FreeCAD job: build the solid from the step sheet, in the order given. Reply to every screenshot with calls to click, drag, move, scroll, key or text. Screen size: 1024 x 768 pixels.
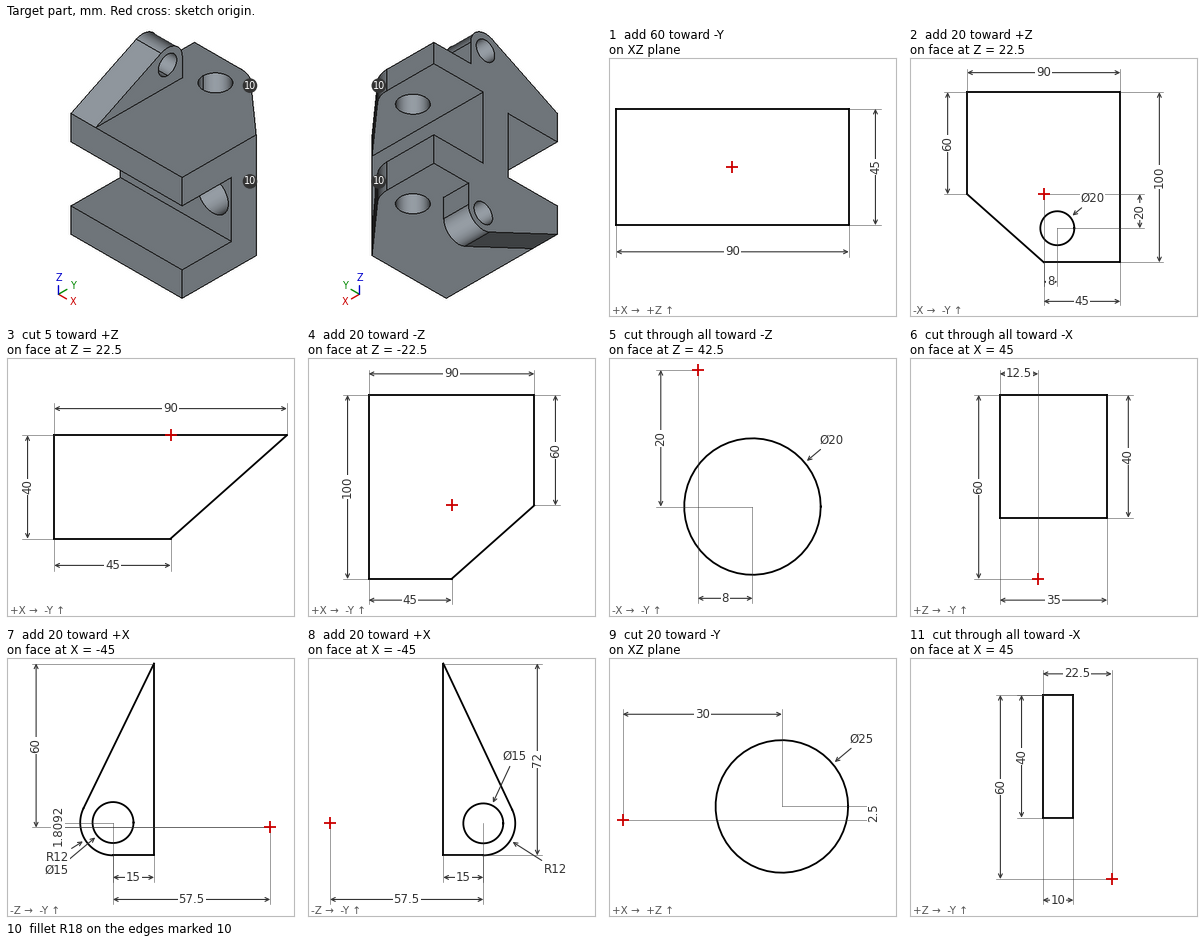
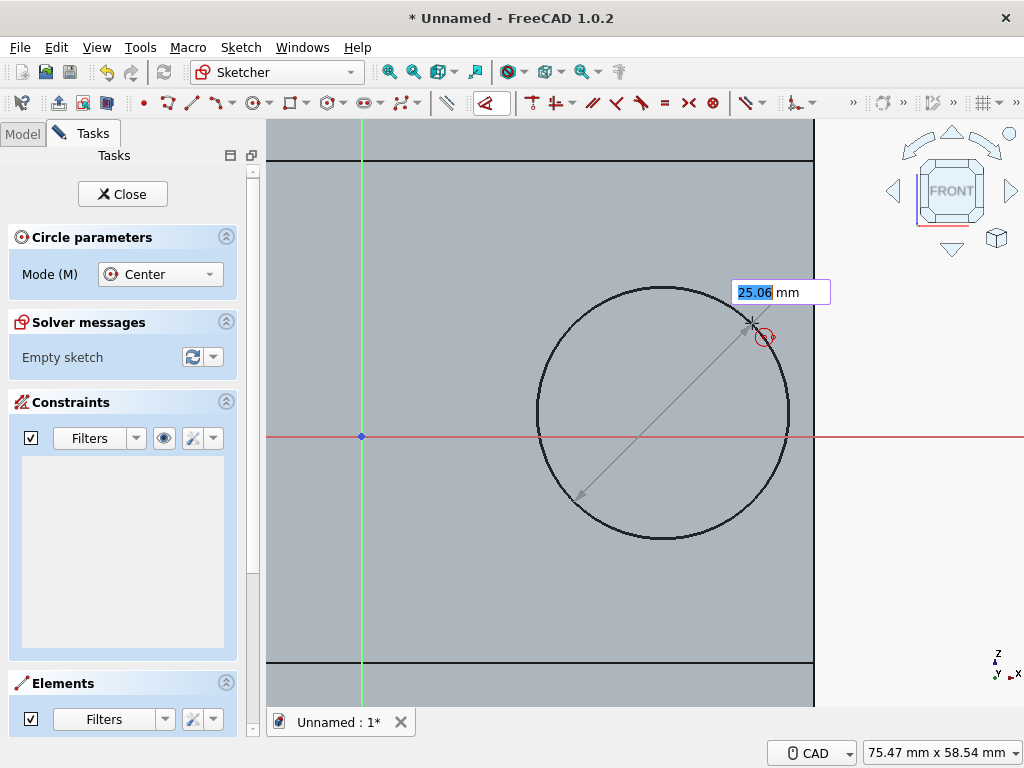
text(25)
key(Return)
key(Escape)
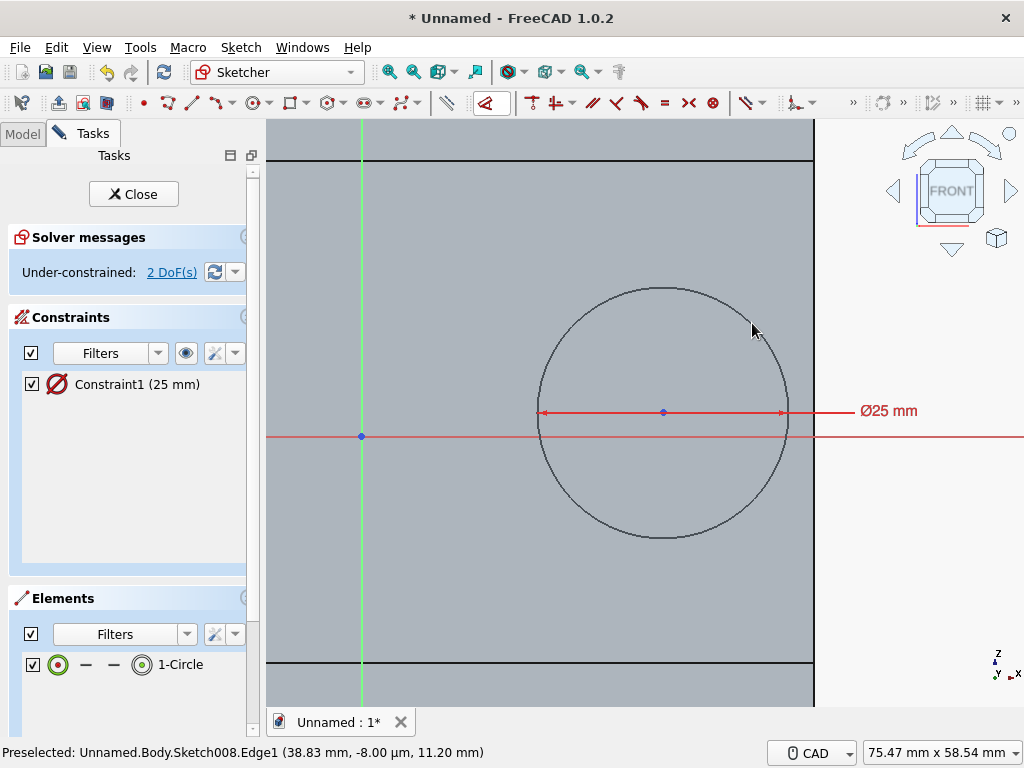
click(663, 413)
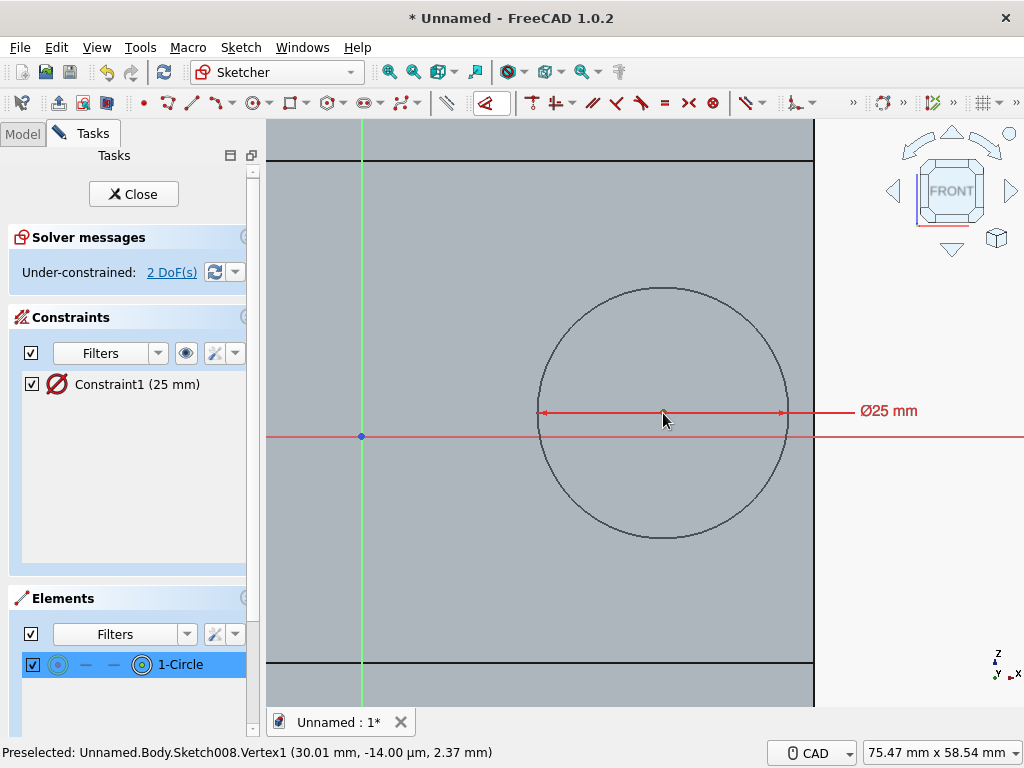
key(l)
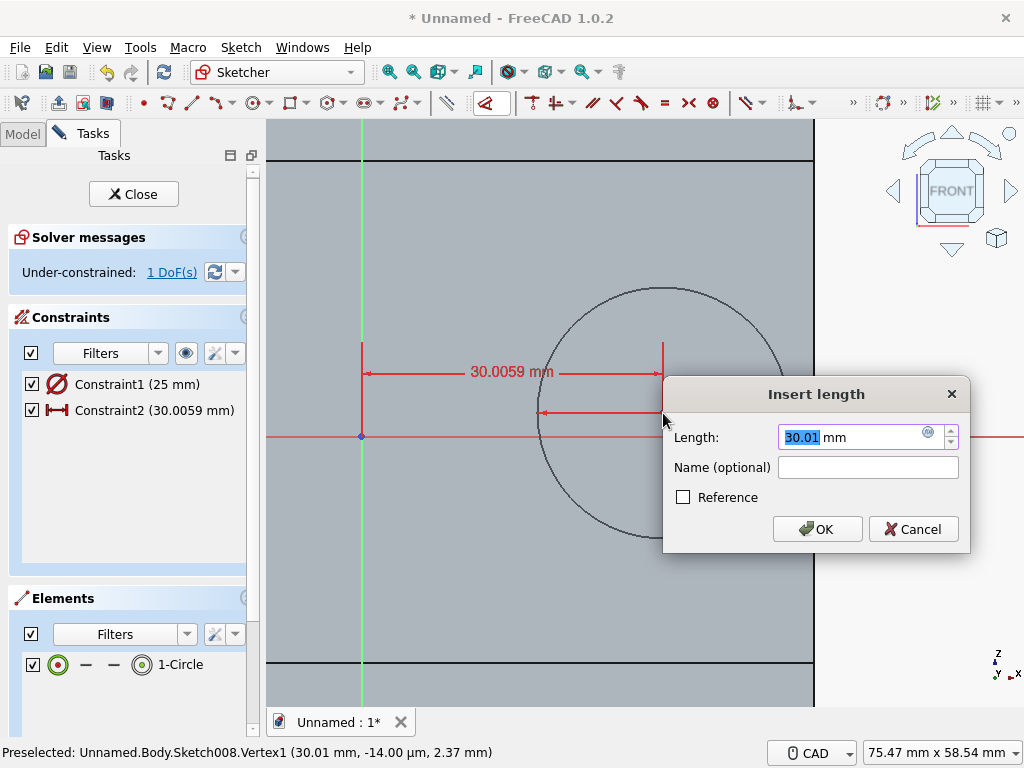
text(30)
key(Return)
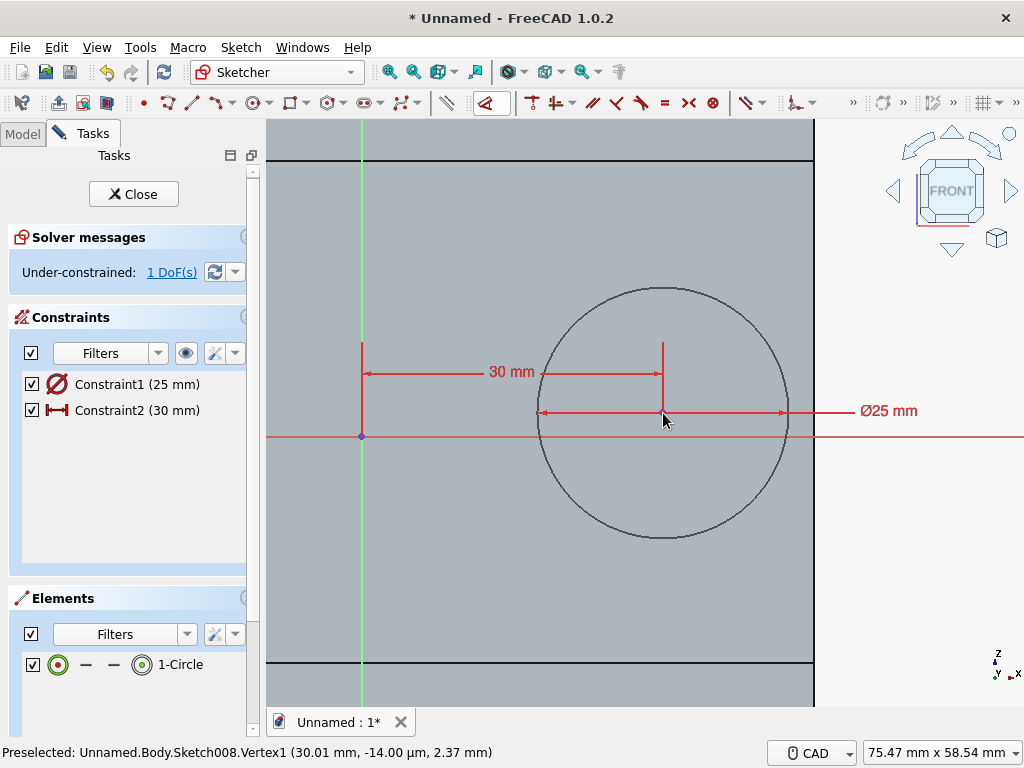
scroll(663, 413, up, 3)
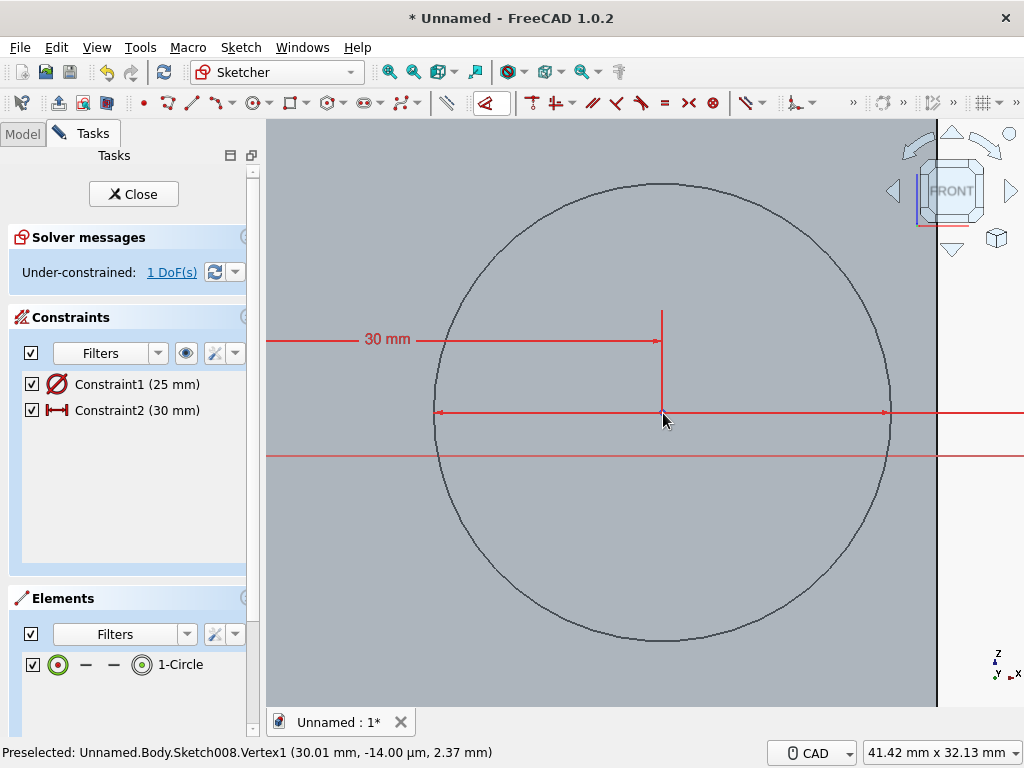
click(662, 413)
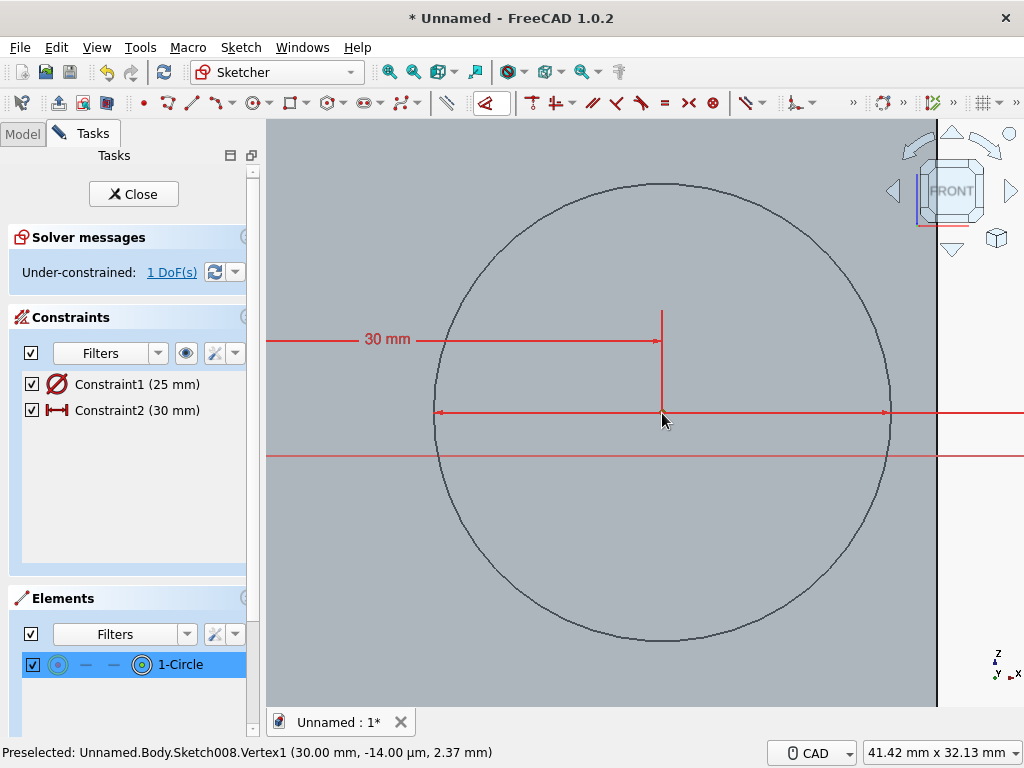
key(i)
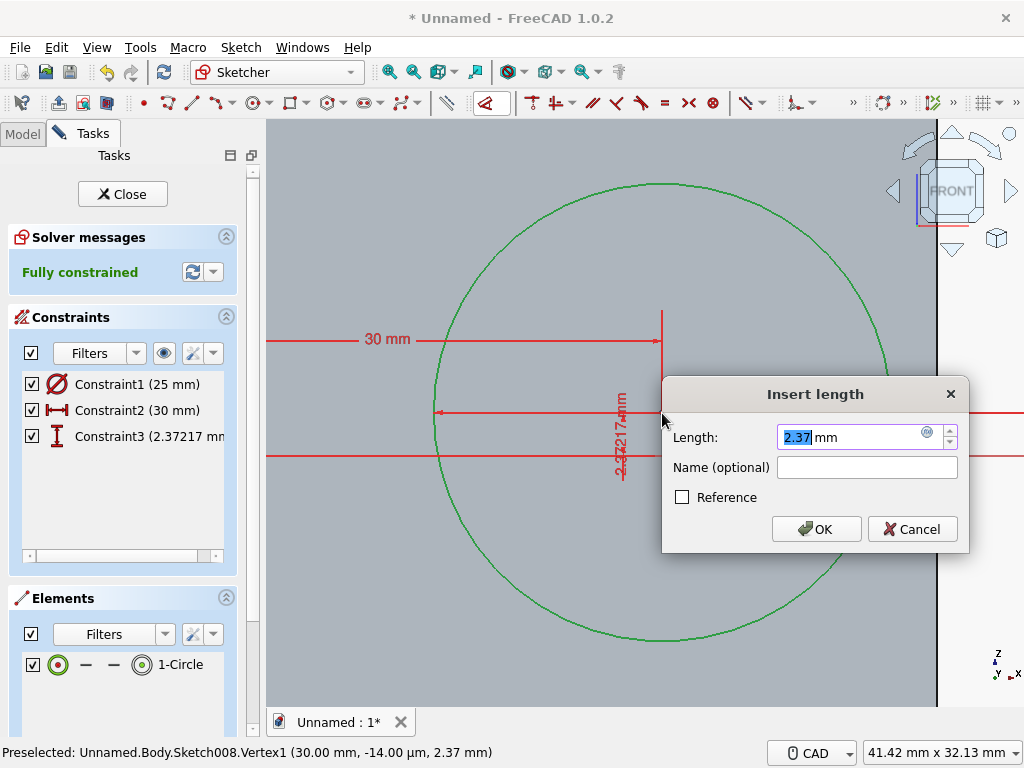
text(2.5)
key(Return)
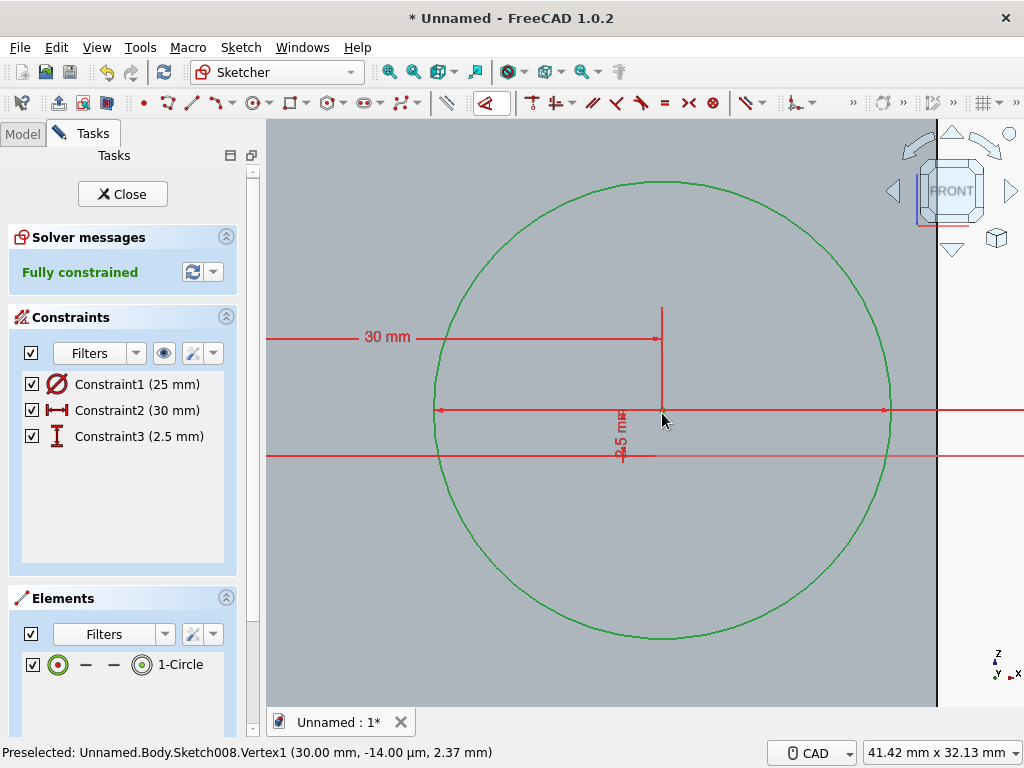
click(123, 194)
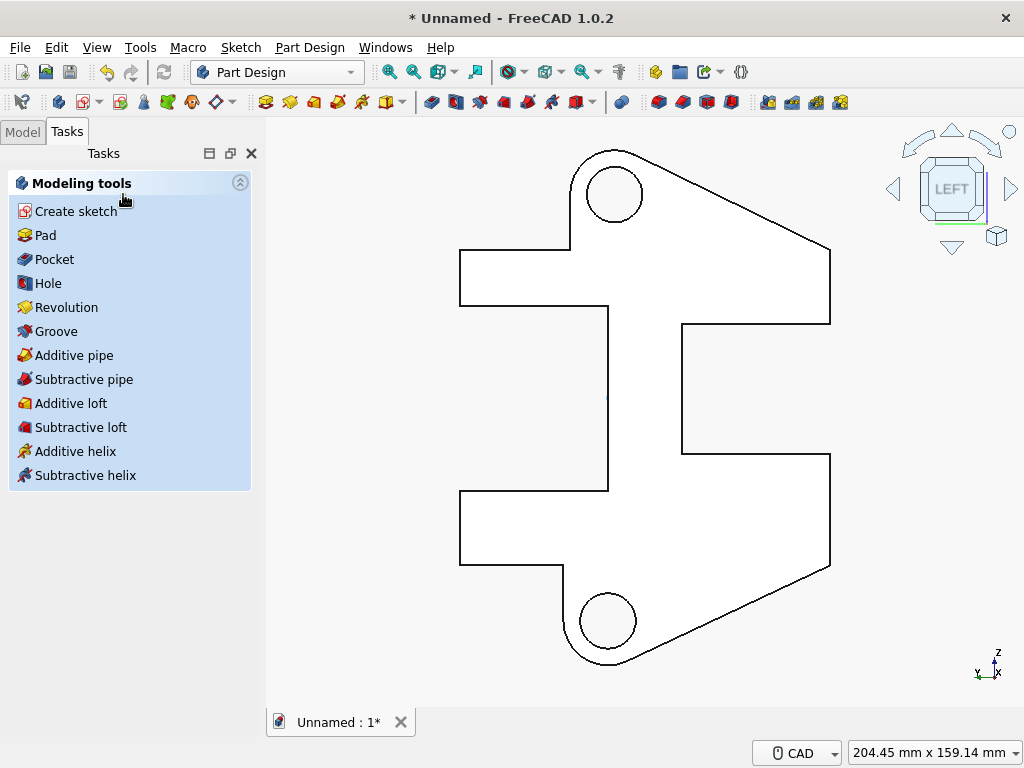
click(432, 102)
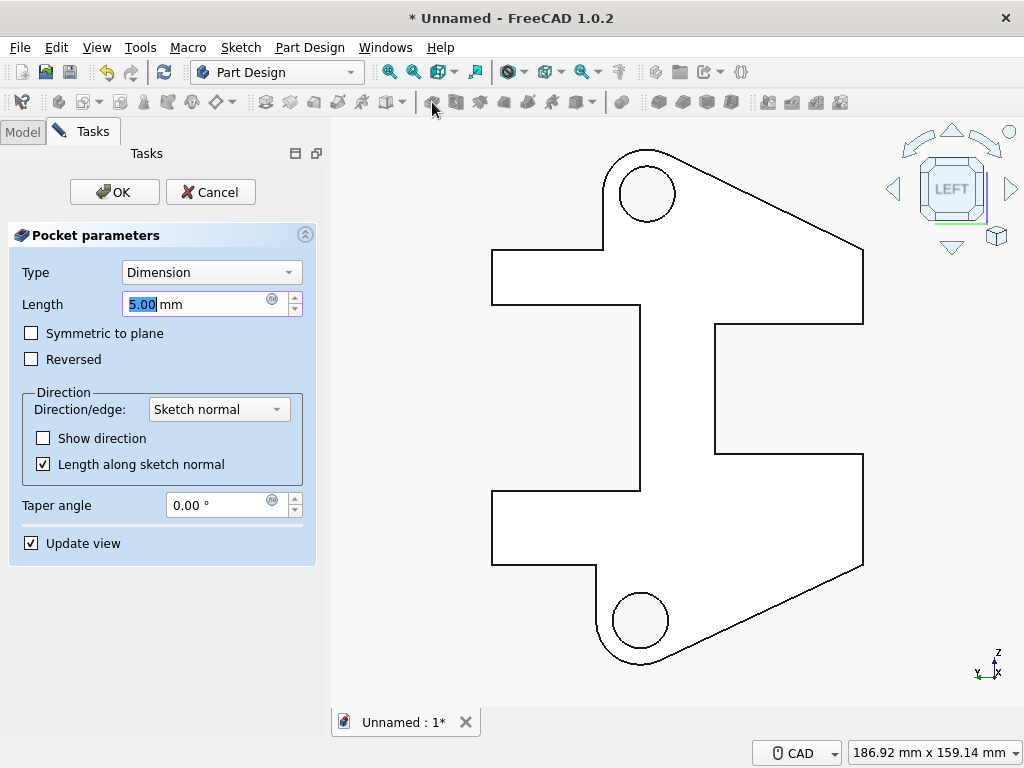
text(20)
key(Tab)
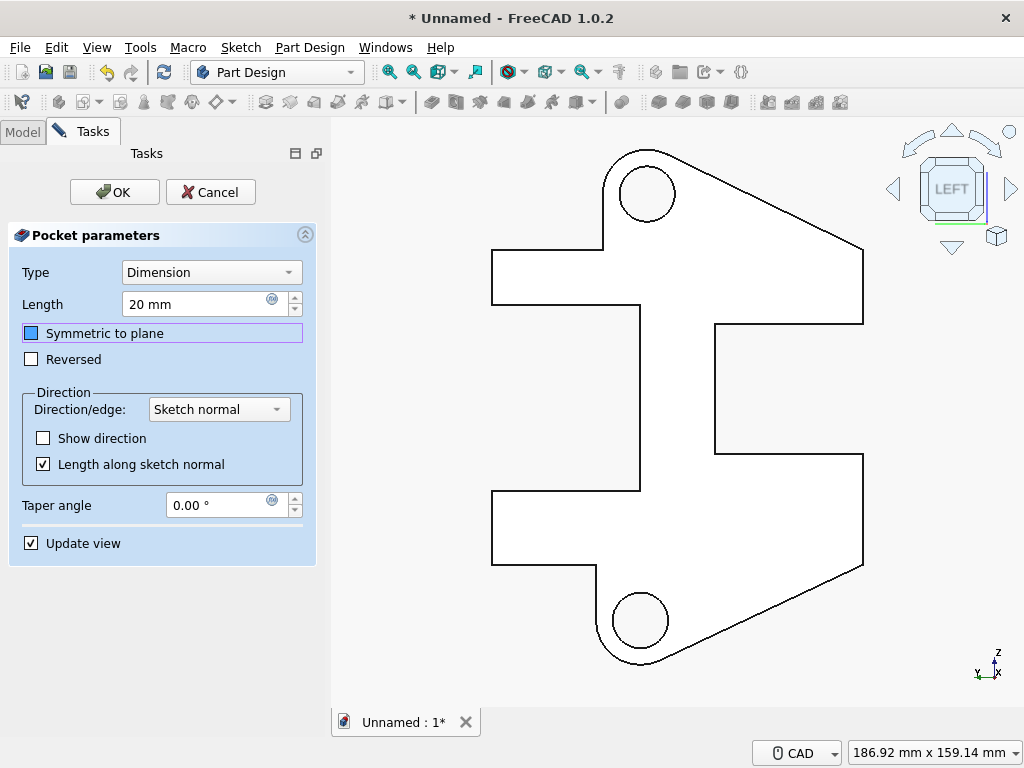
click(30, 359)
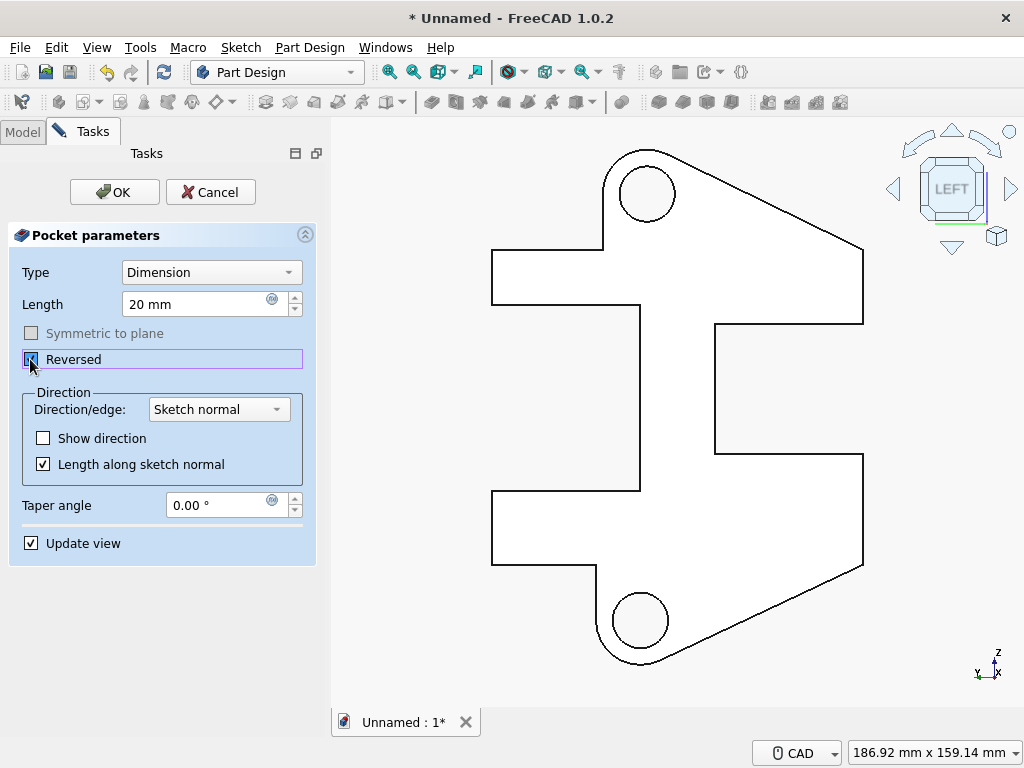
click(115, 192)